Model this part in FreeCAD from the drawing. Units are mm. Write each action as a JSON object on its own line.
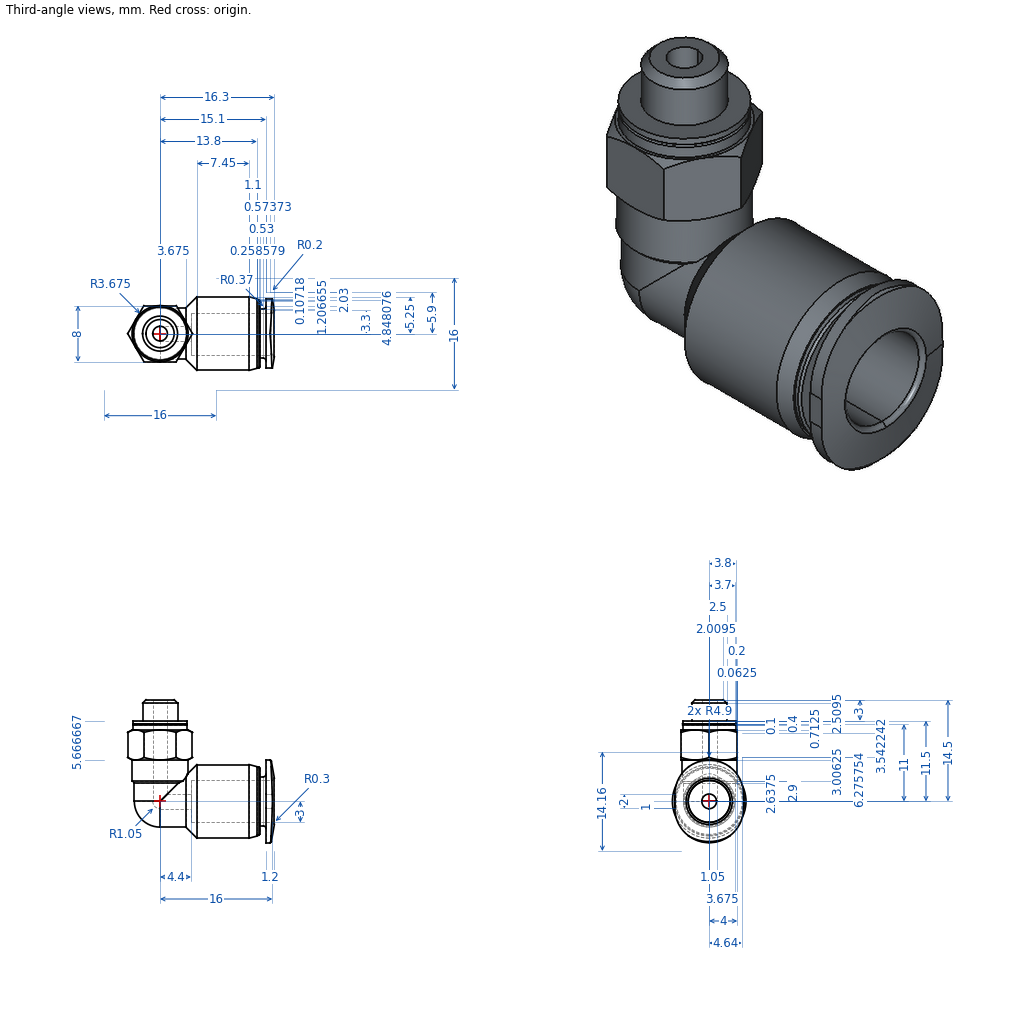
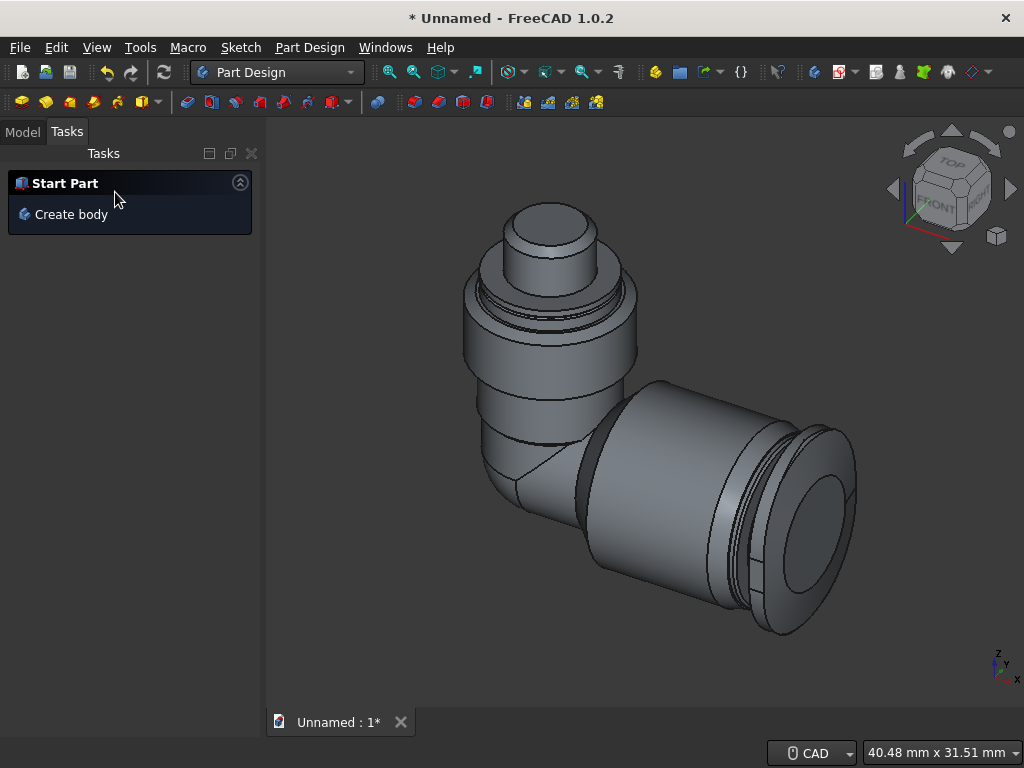
{"action": "left_click", "coordinate": [840, 72]}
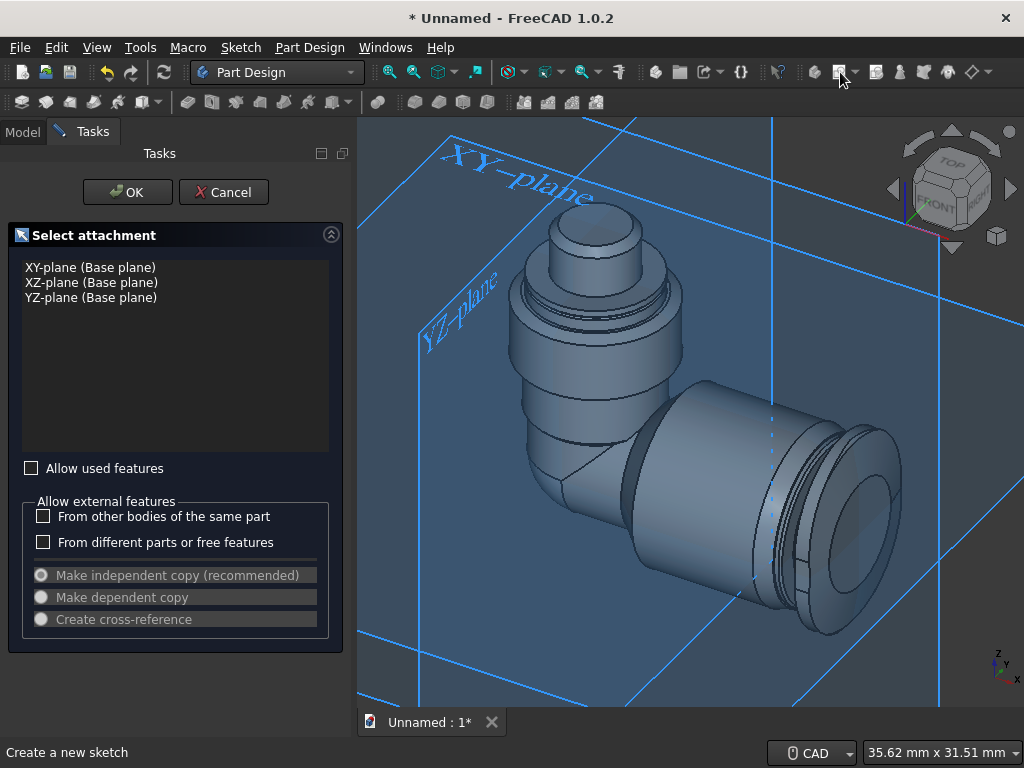
{"action": "left_click", "coordinate": [82, 298]}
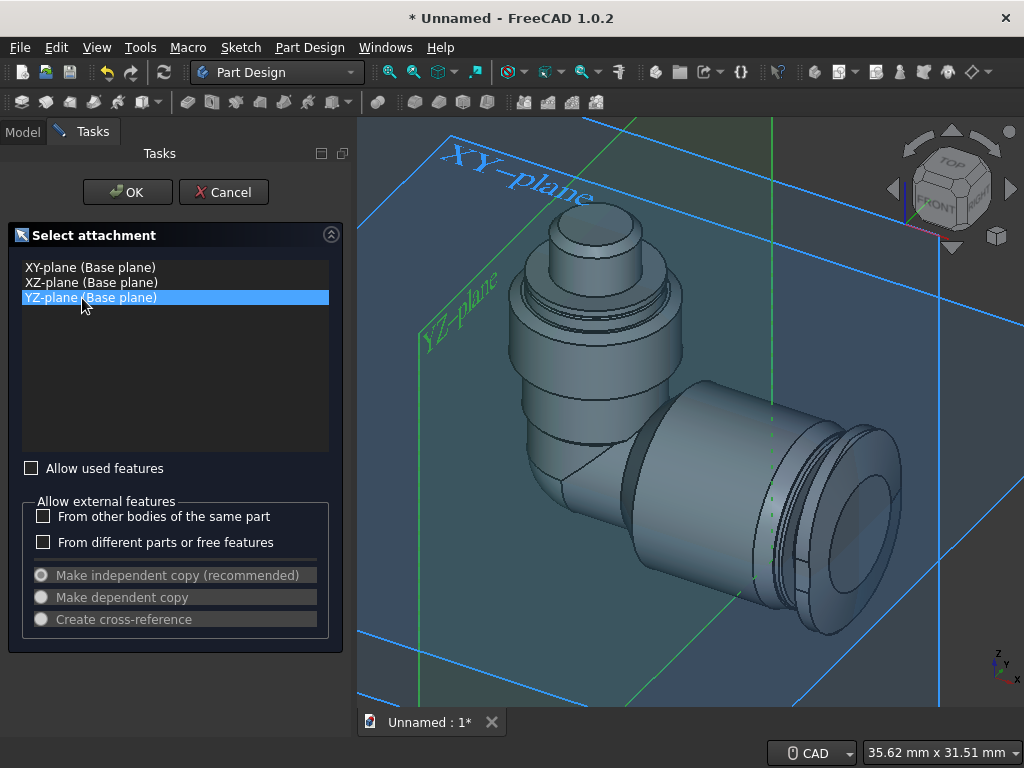
{"action": "left_click", "coordinate": [128, 192]}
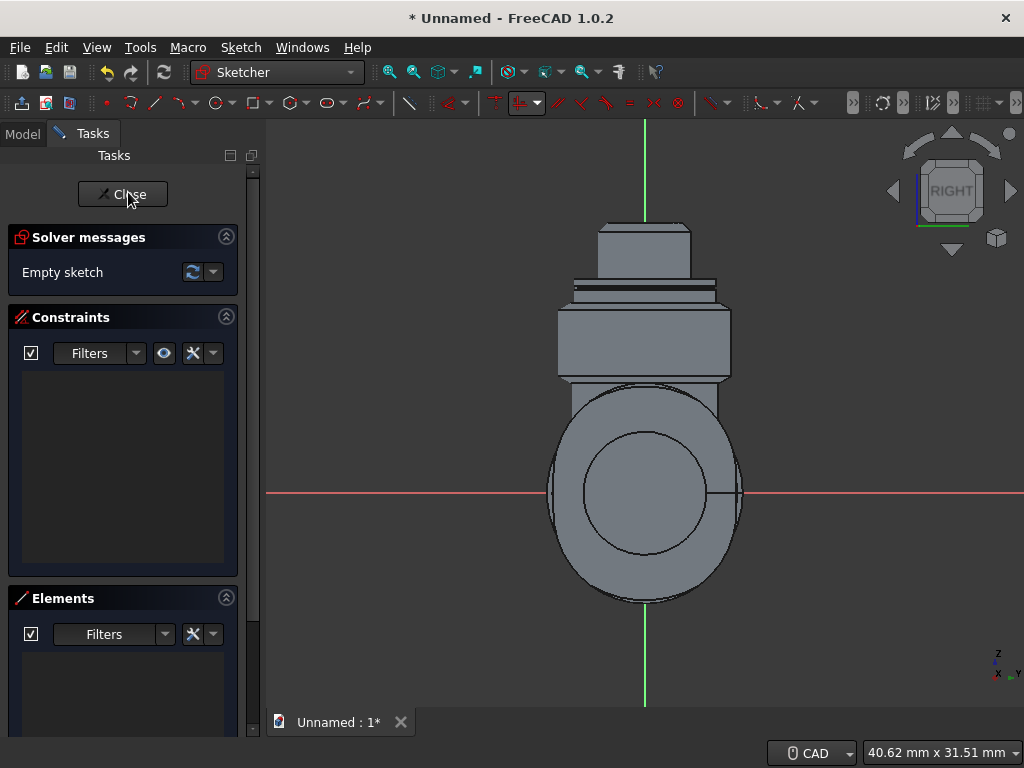
{"action": "left_click", "coordinate": [70, 104]}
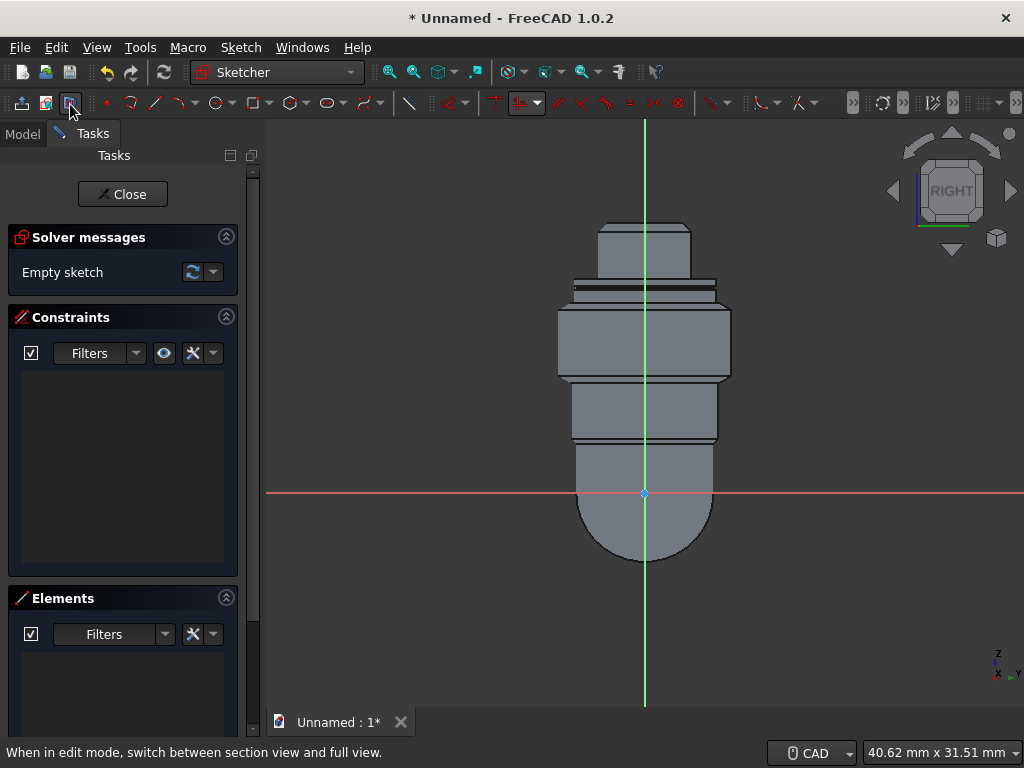
{"action": "scroll", "coordinate": [814, 246], "scroll_direction": "up", "scroll_amount": 2}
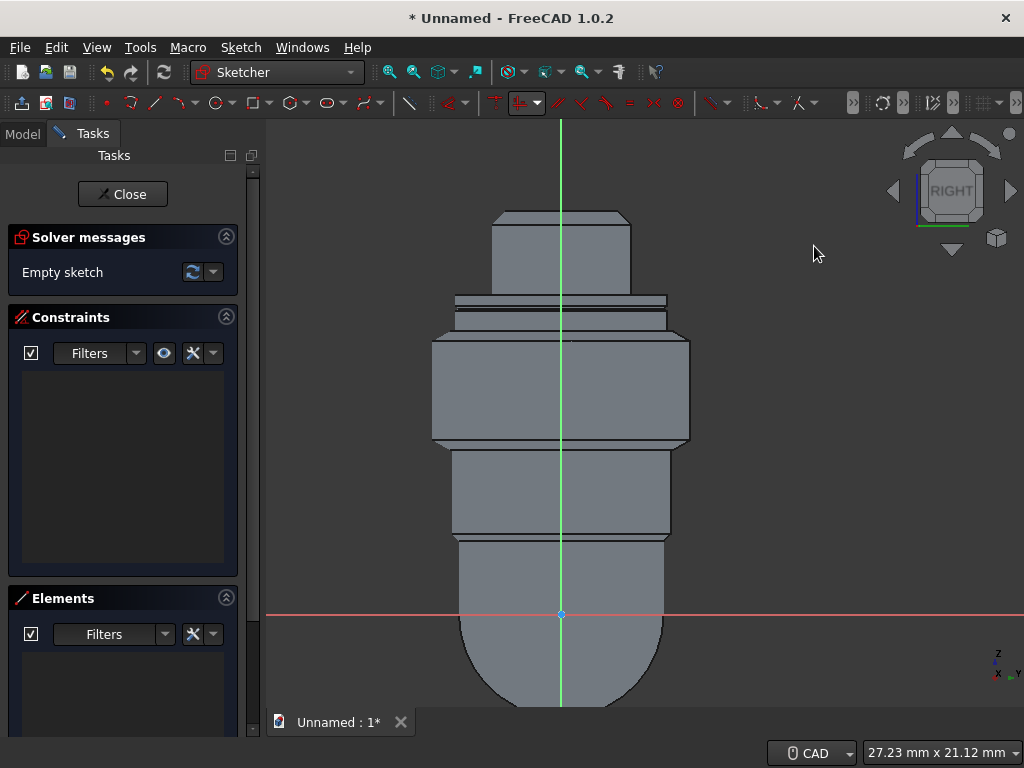
{"action": "left_click", "coordinate": [254, 104]}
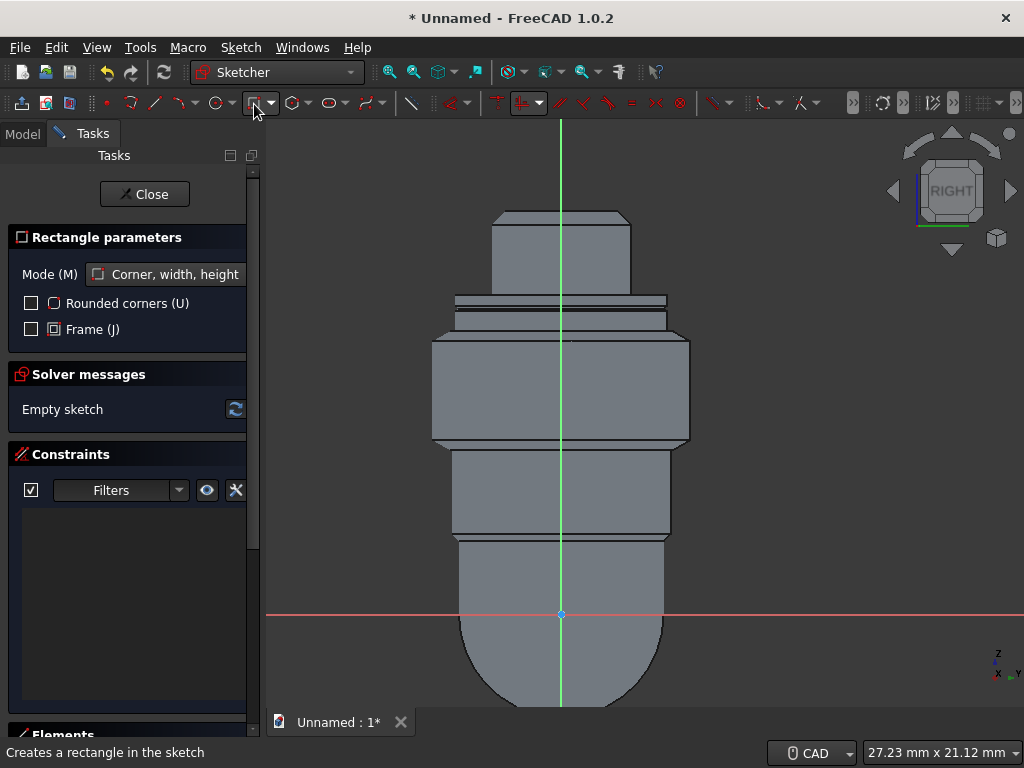
{"action": "left_click", "coordinate": [561, 615]}
{"action": "left_click", "coordinate": [591, 211]}
{"action": "key", "text": "Escape"}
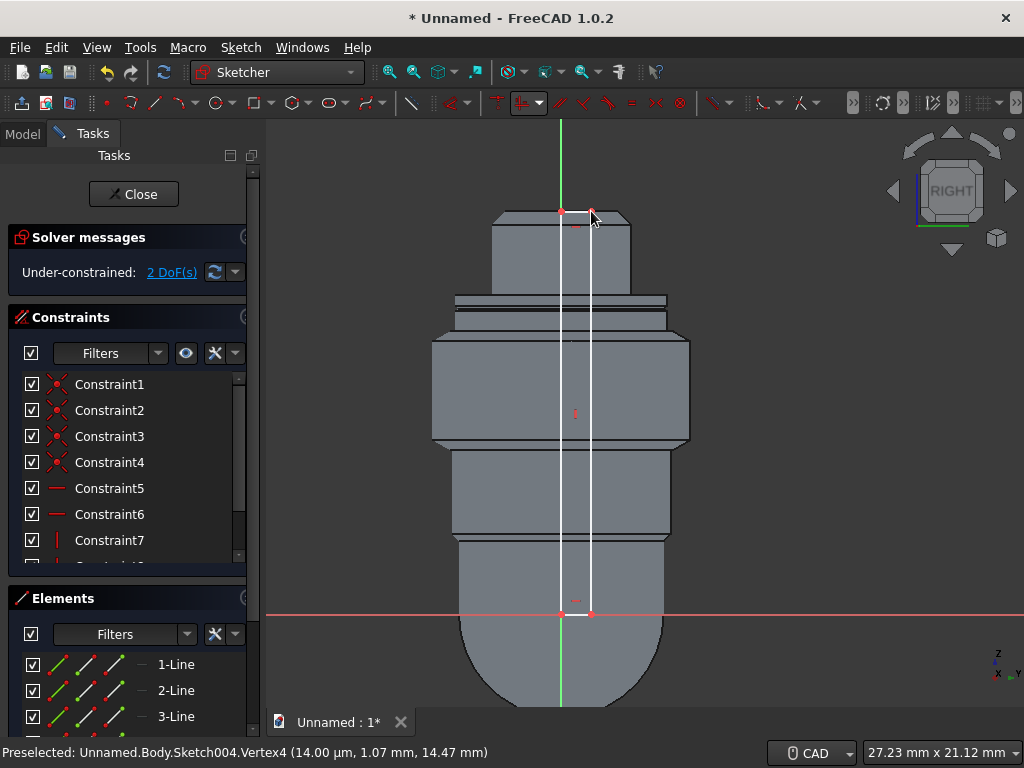
{"action": "left_click", "coordinate": [450, 104]}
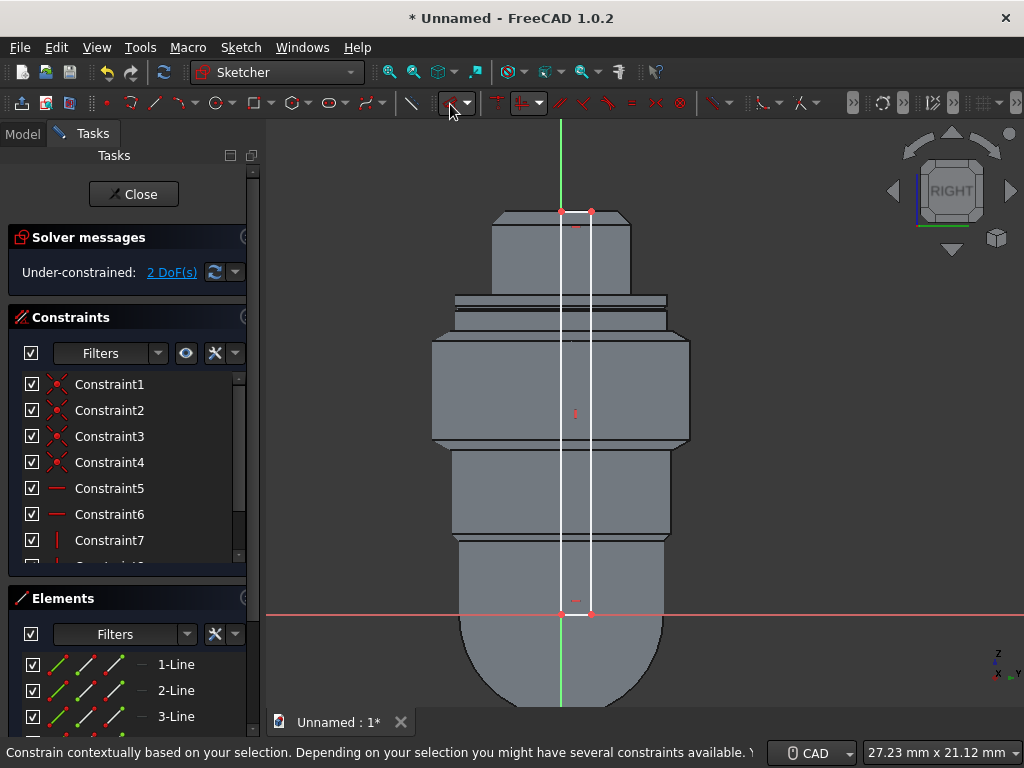
{"action": "scroll", "coordinate": [573, 615], "scroll_direction": "up", "scroll_amount": 2}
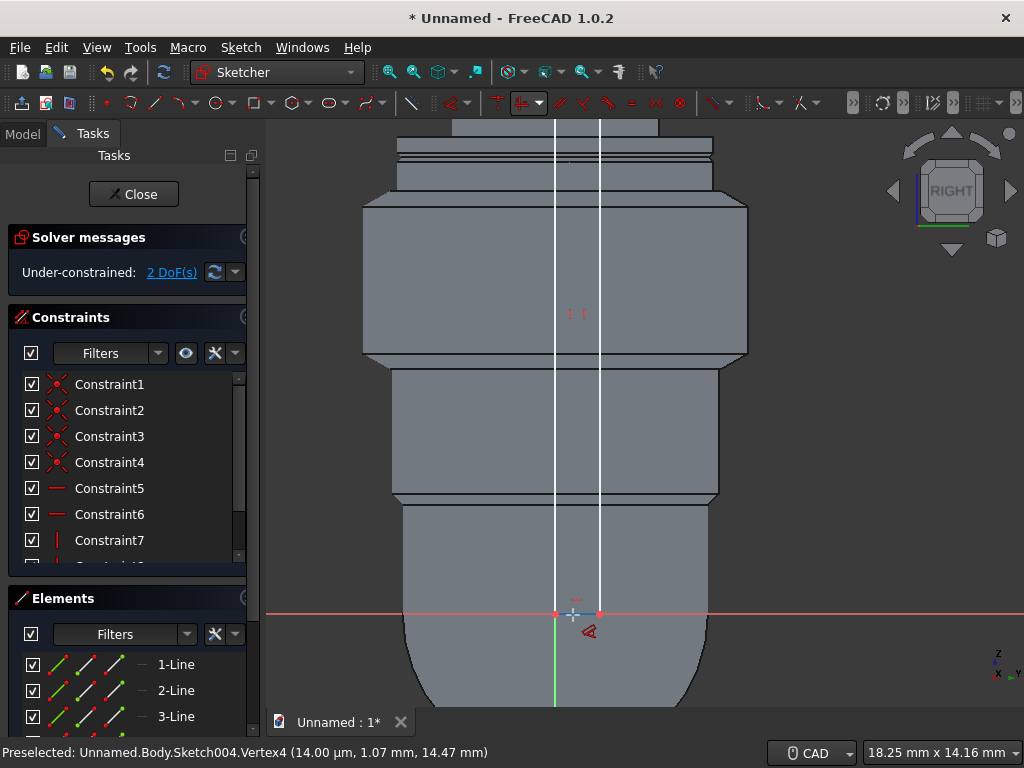
{"action": "left_click", "coordinate": [573, 614]}
{"action": "left_click", "coordinate": [577, 648]}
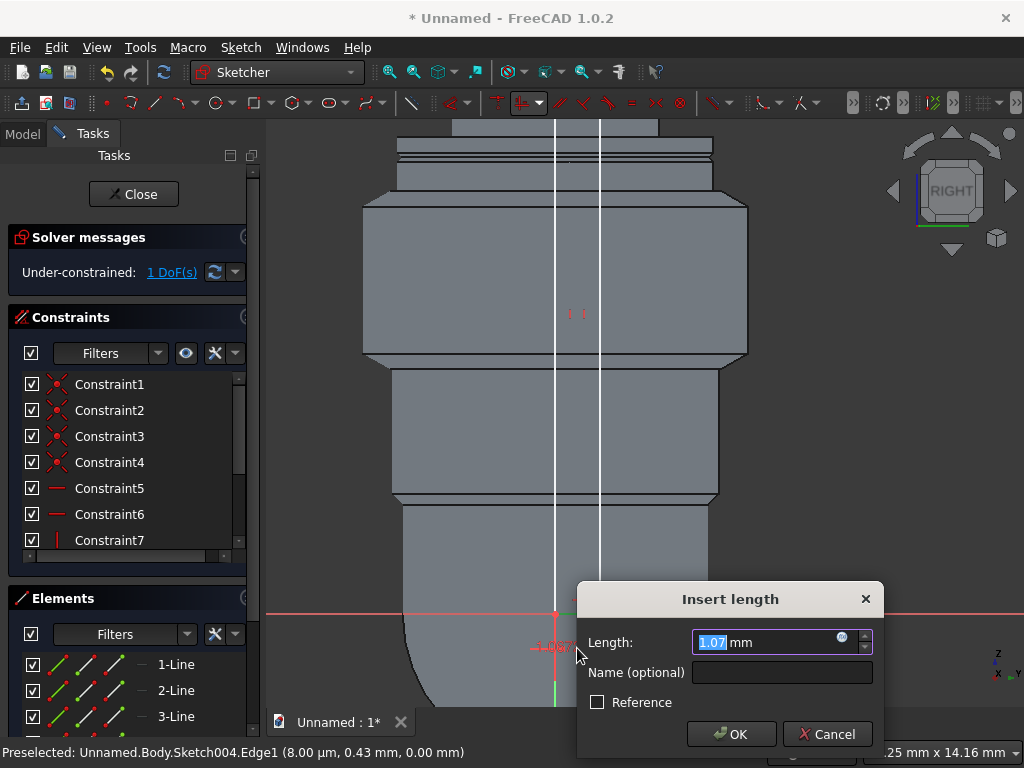
{"action": "type", "text": "1.05"}
{"action": "key", "text": "Return"}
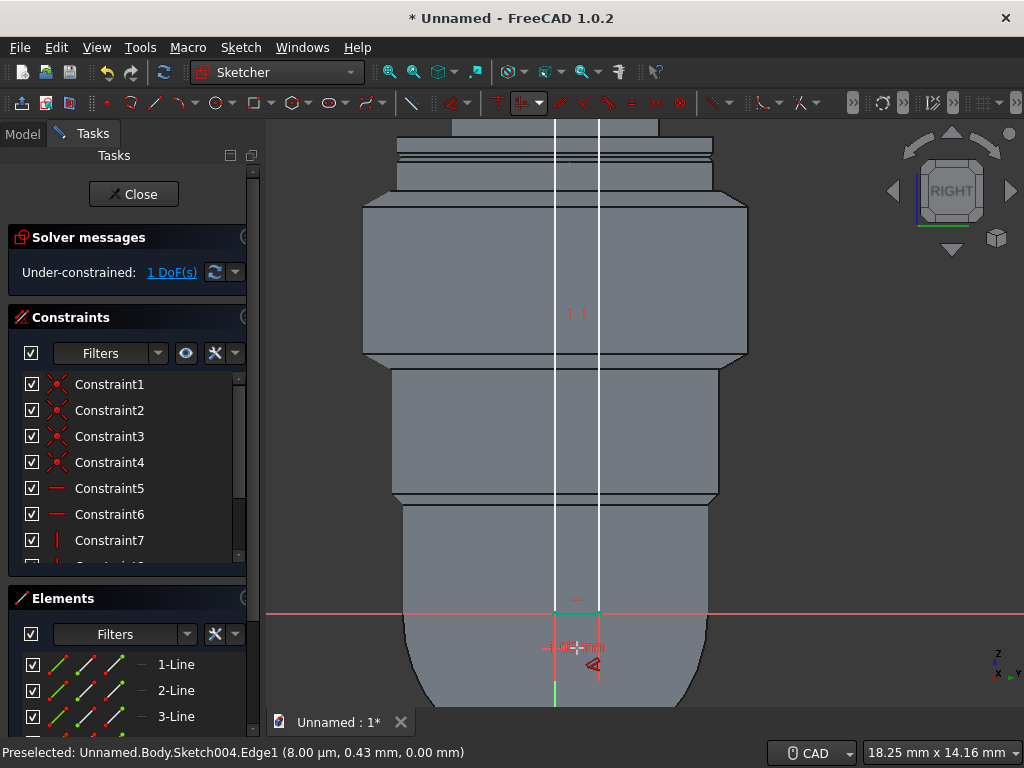
{"action": "left_click", "coordinate": [599, 434]}
{"action": "left_click", "coordinate": [633, 381]}